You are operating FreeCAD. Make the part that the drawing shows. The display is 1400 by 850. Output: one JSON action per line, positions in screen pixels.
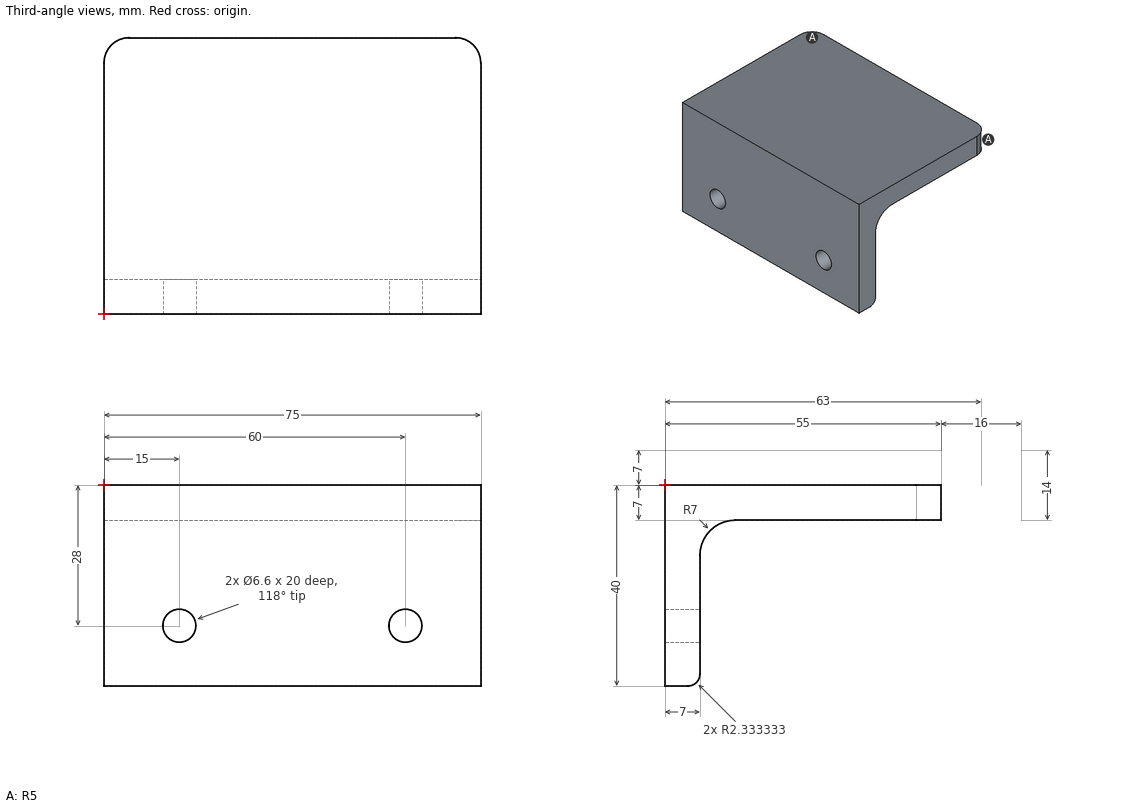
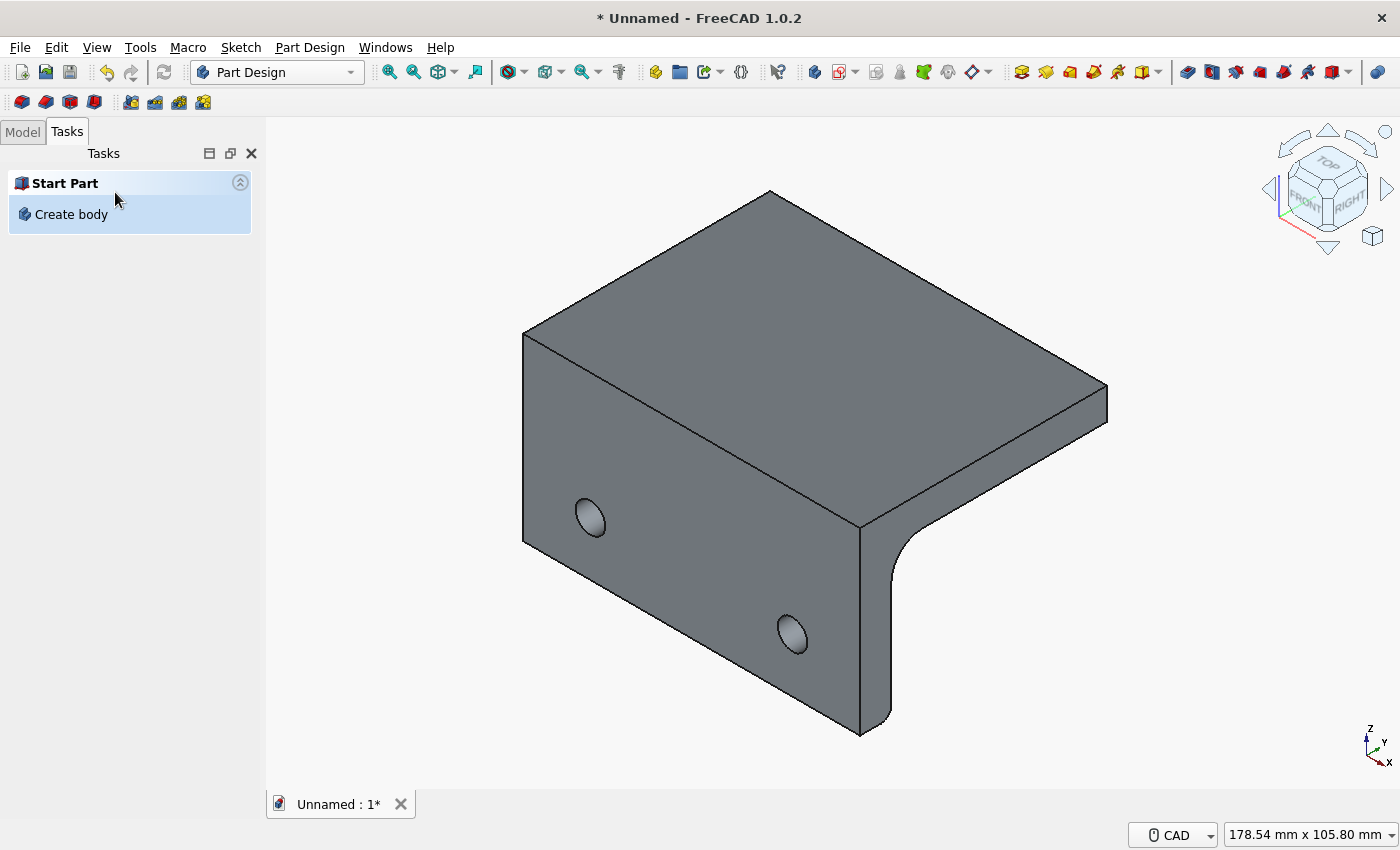
{"action": "key", "text": "2"}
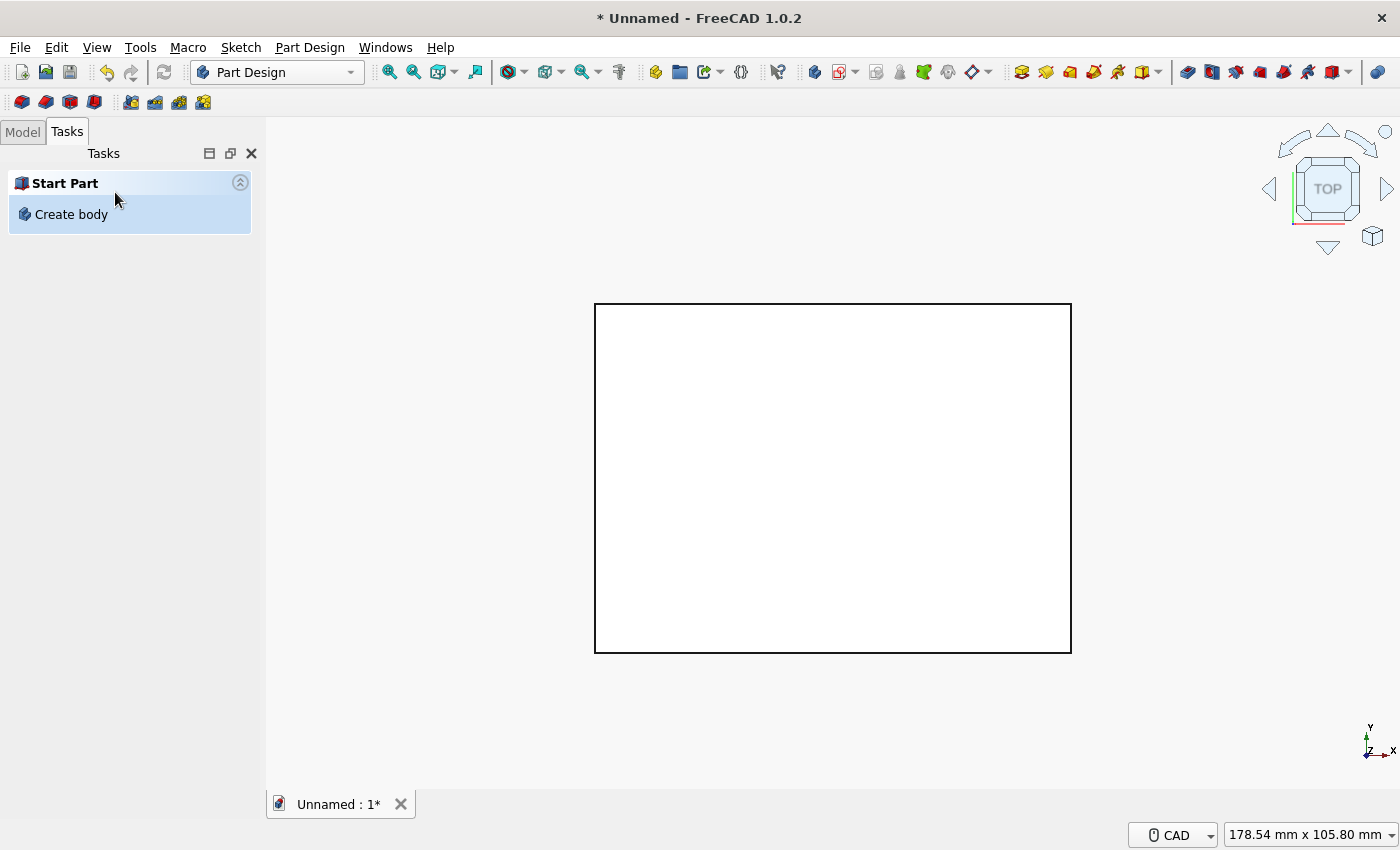
{"action": "key", "text": "1"}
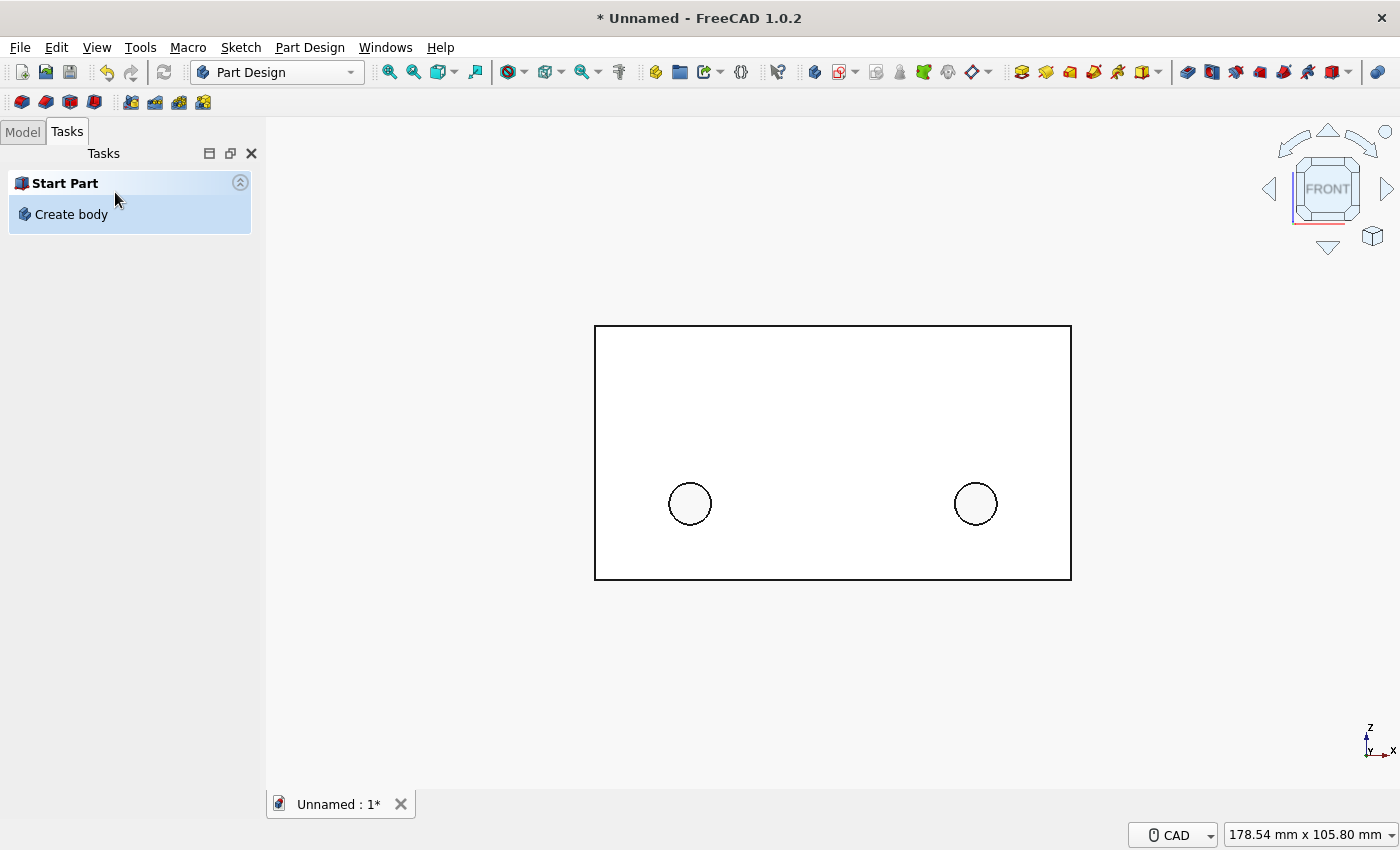
{"action": "key", "text": "v f"}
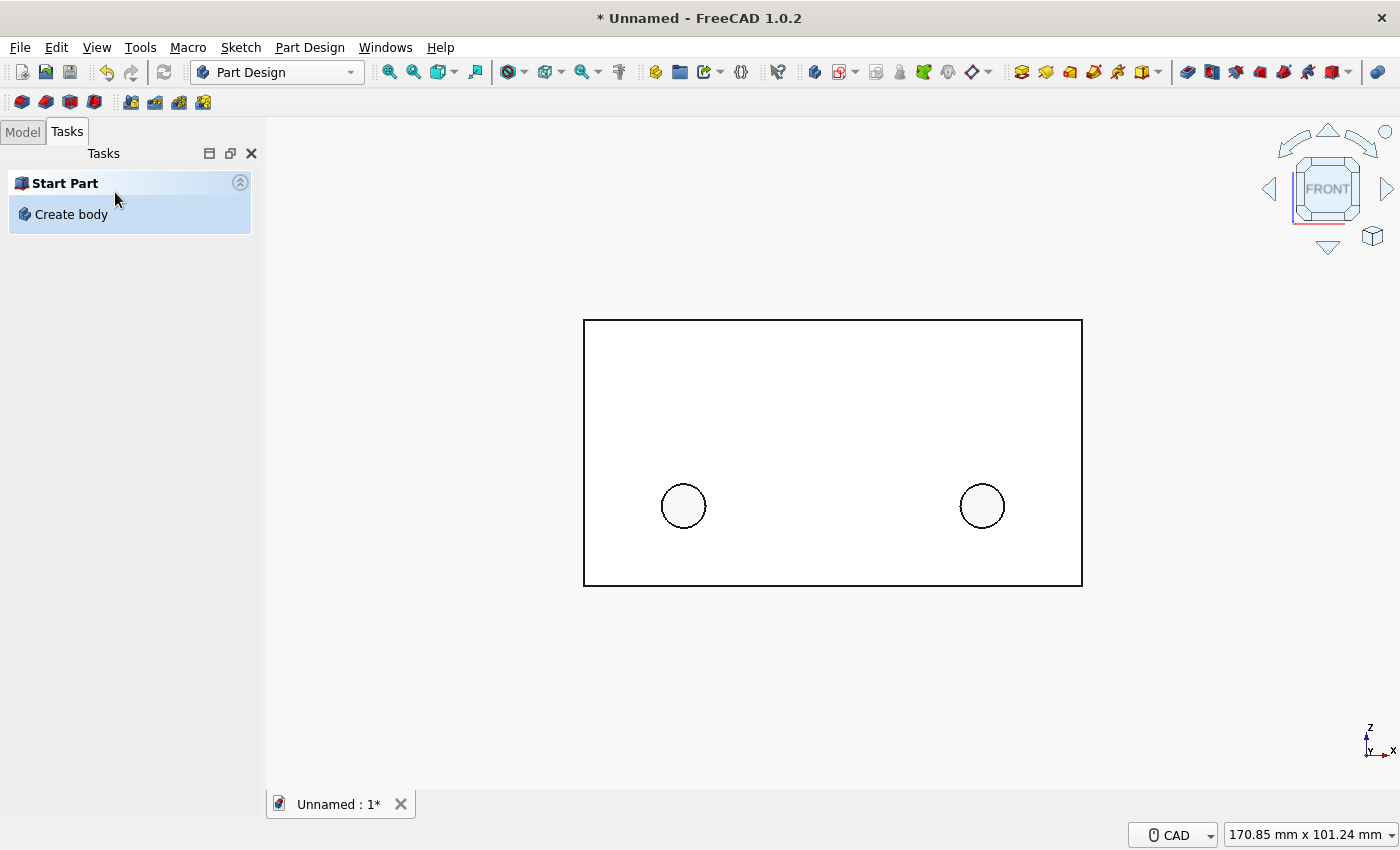
{"action": "key", "text": "3"}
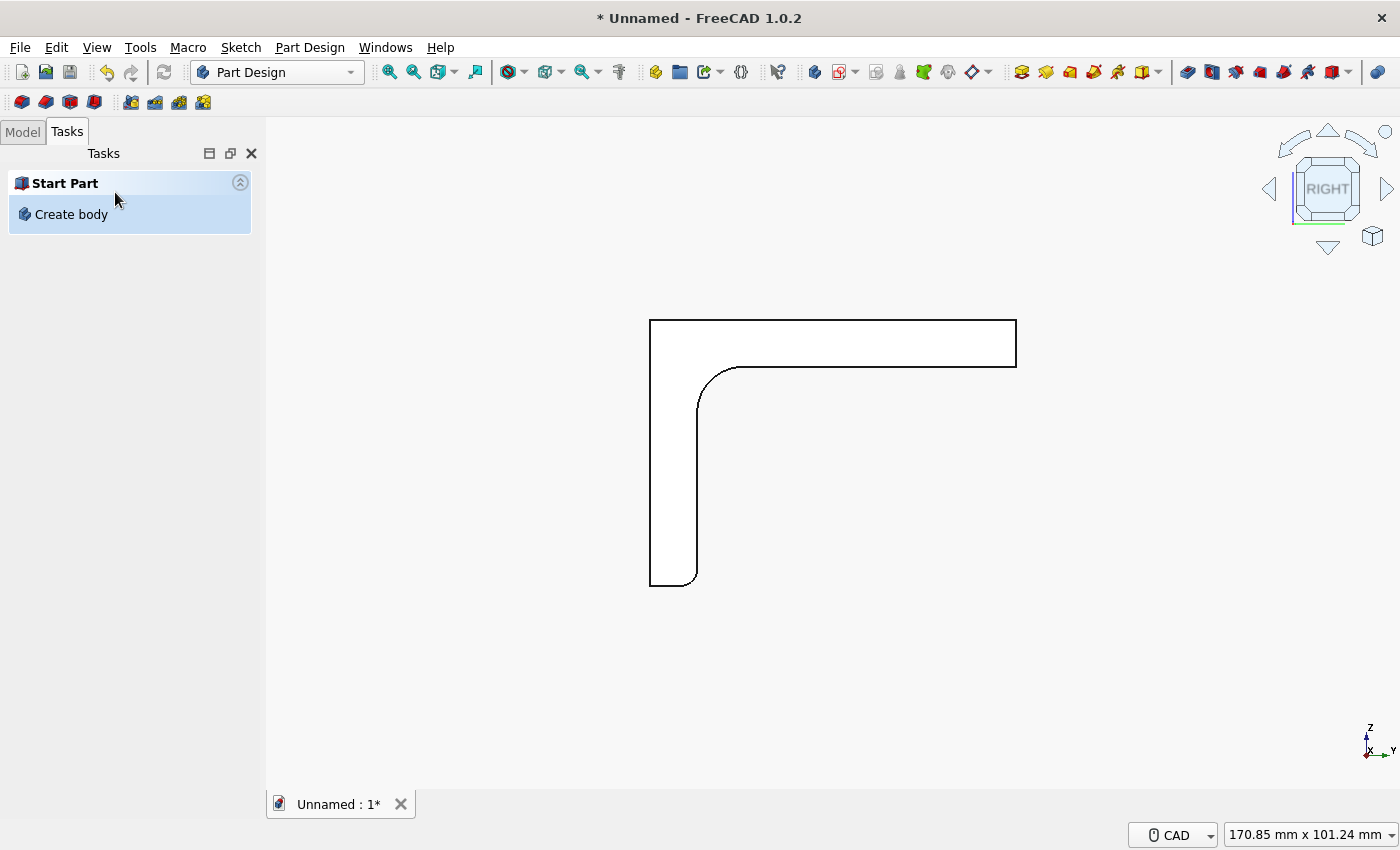
{"action": "left_click", "coordinate": [390, 72]}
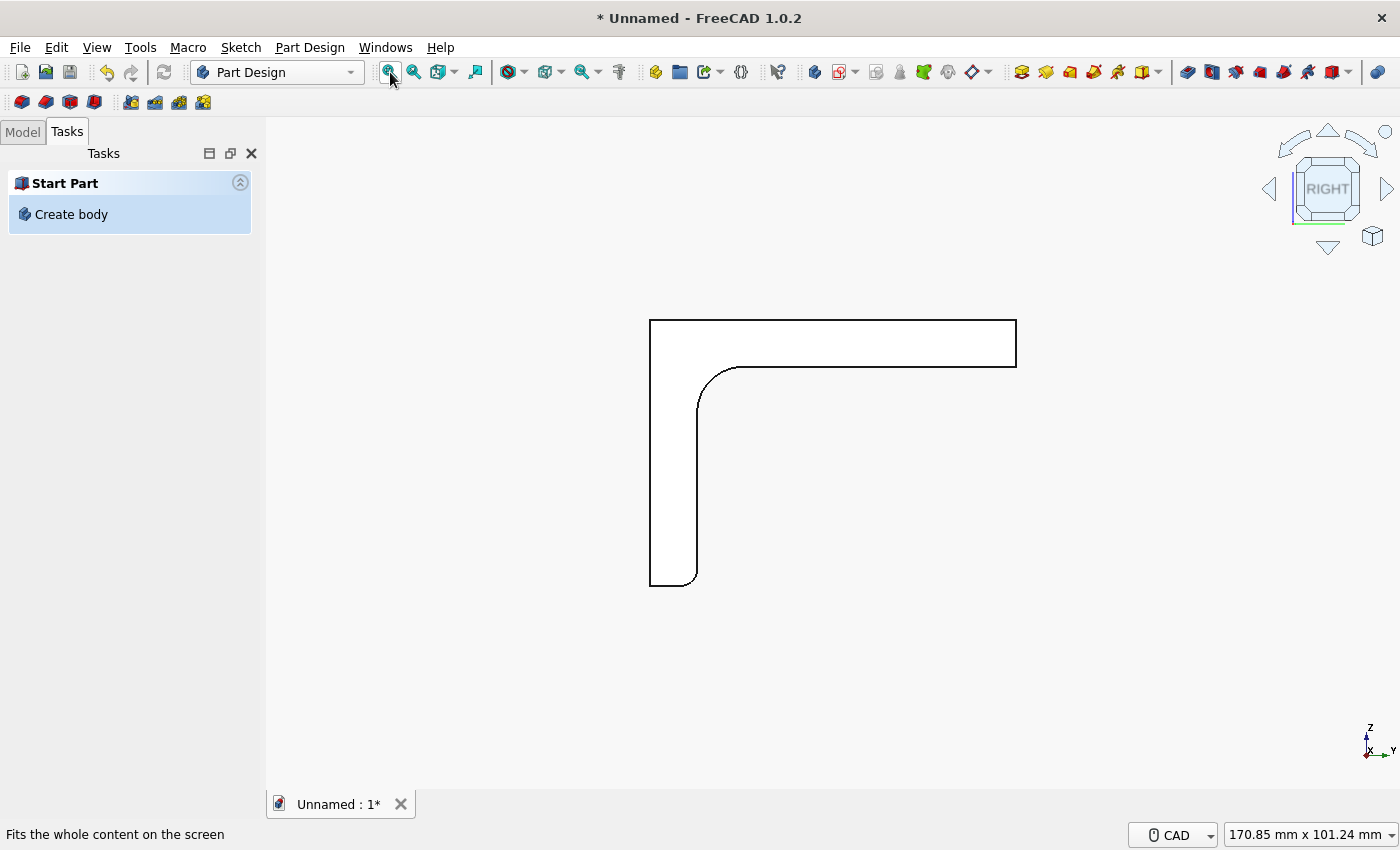
{"action": "left_click", "coordinate": [1016, 342]}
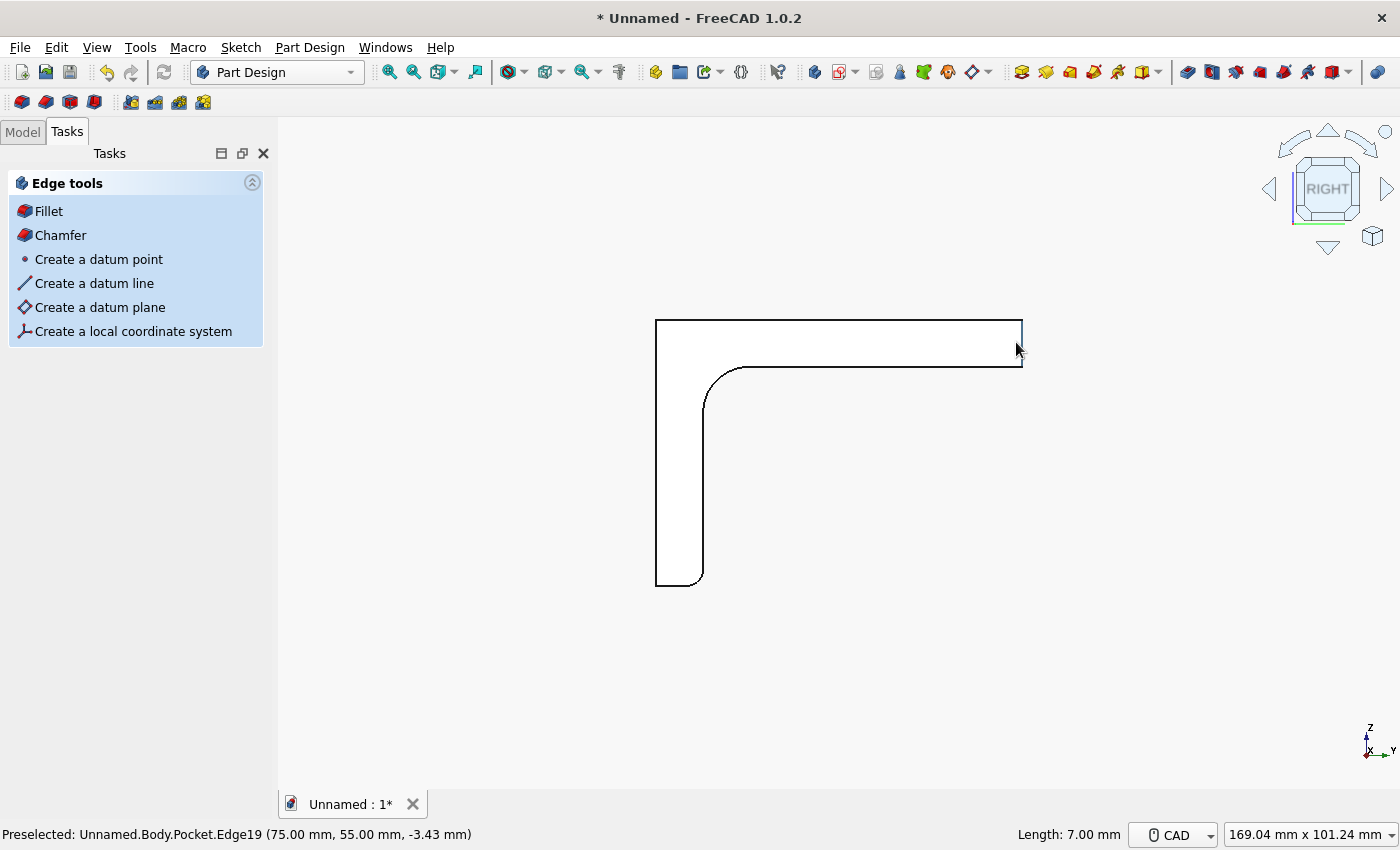
{"action": "key", "text": "5"}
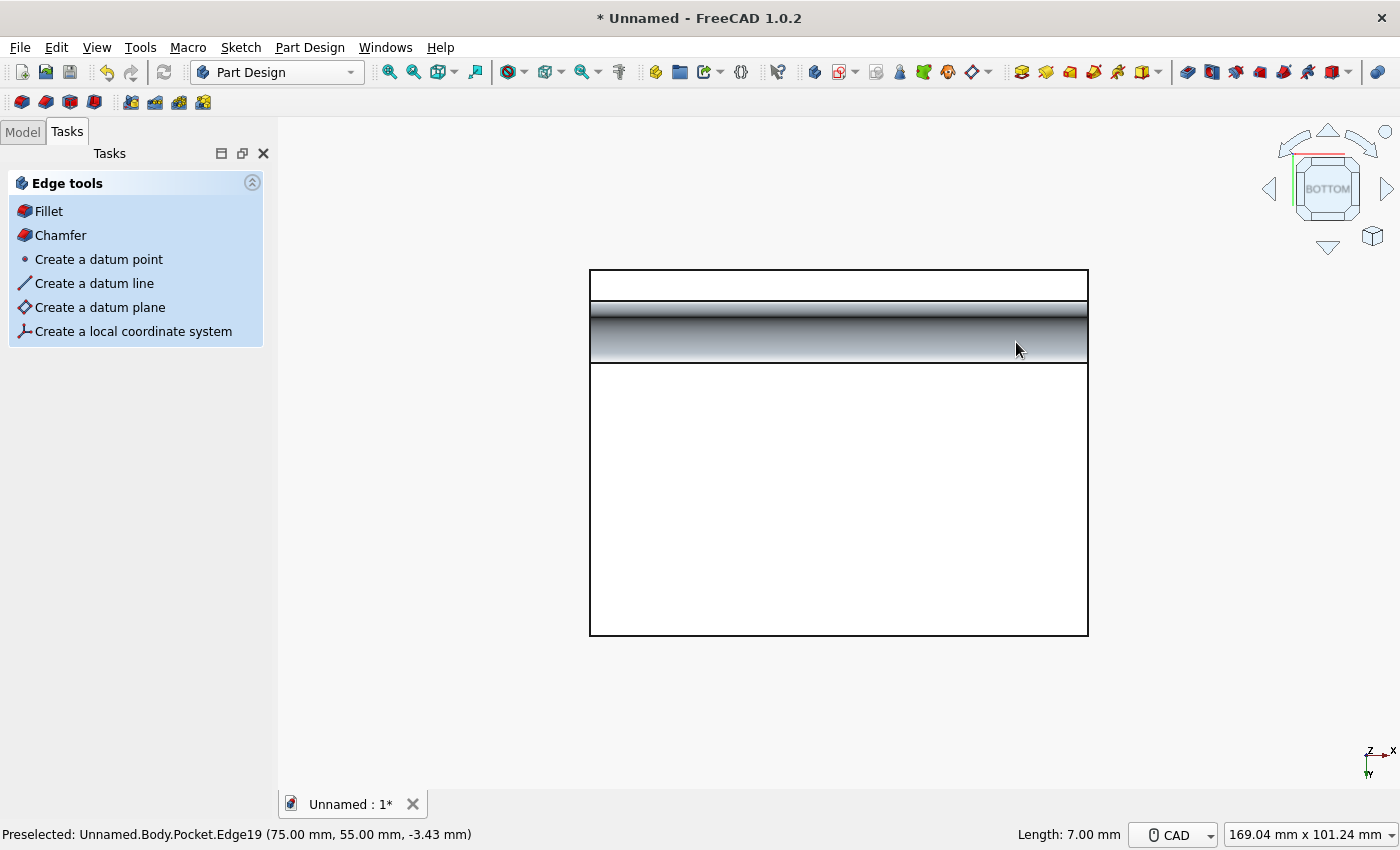
{"action": "key", "text": "4"}